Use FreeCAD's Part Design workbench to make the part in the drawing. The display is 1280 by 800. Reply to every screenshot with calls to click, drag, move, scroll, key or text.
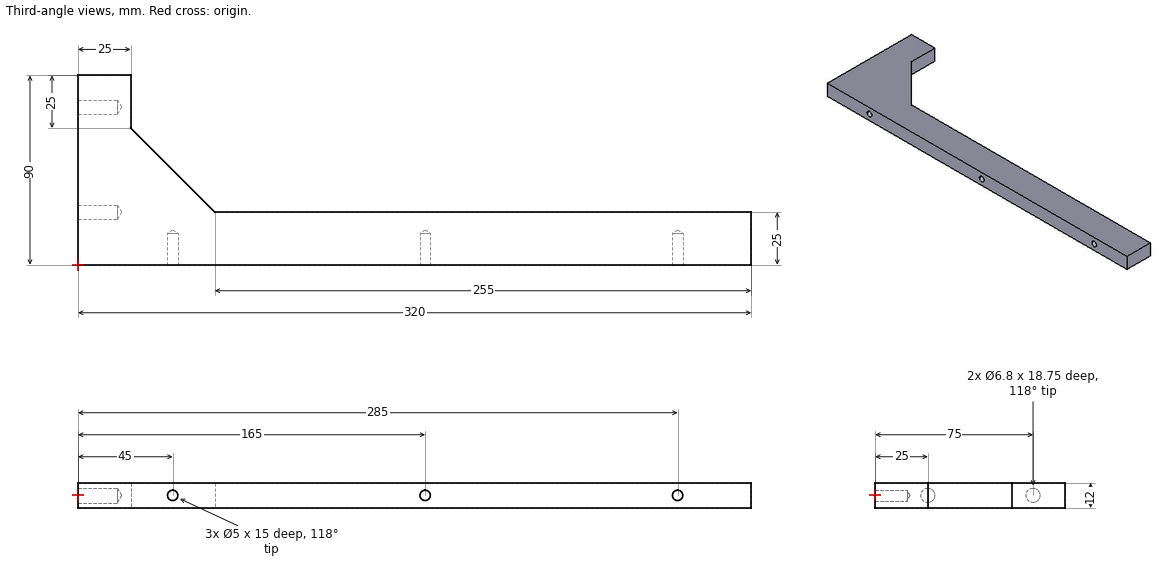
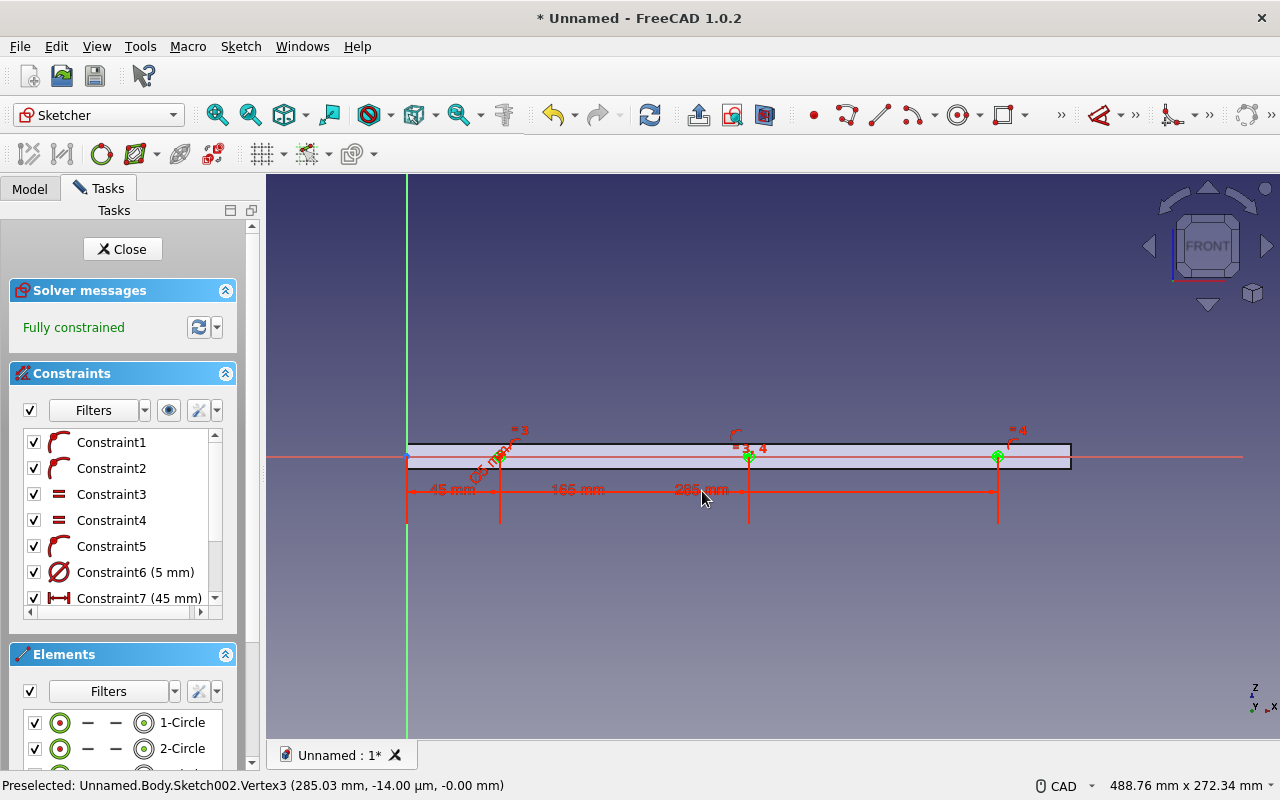
click(123, 249)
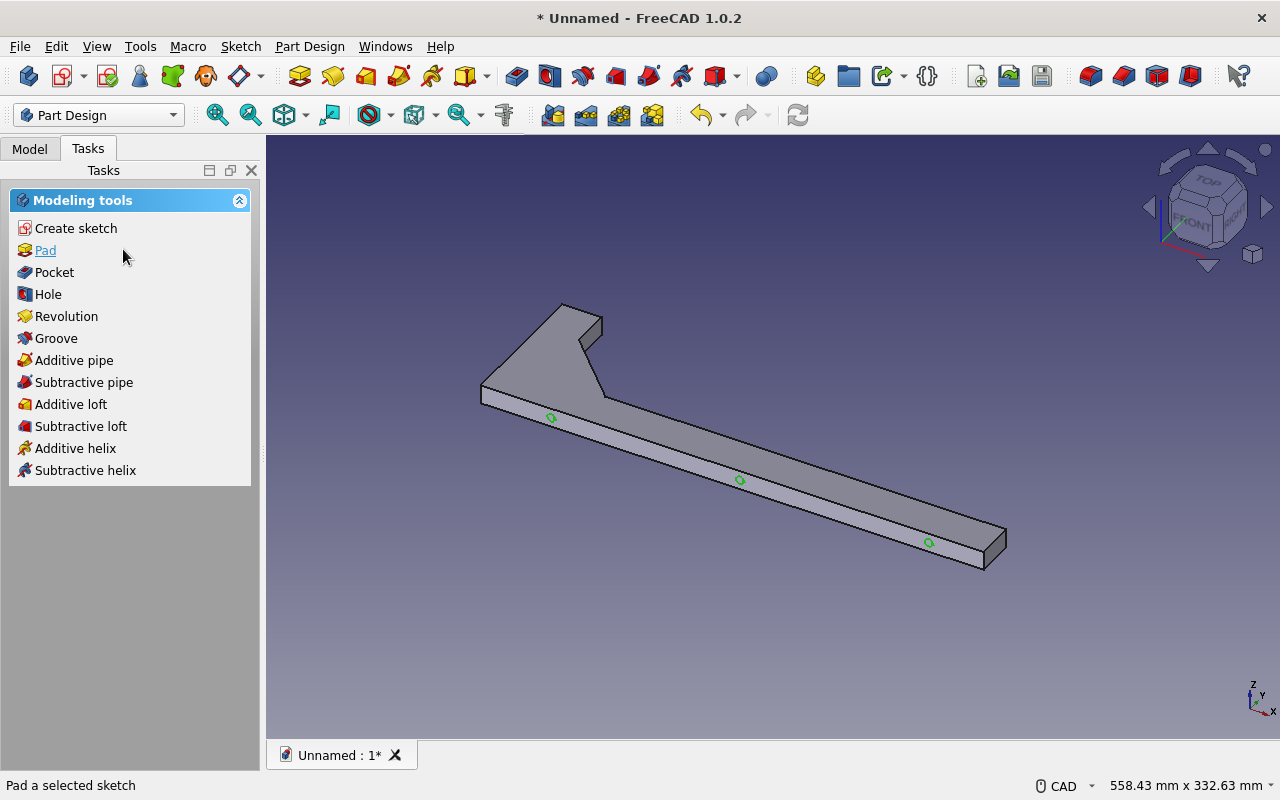
click(550, 76)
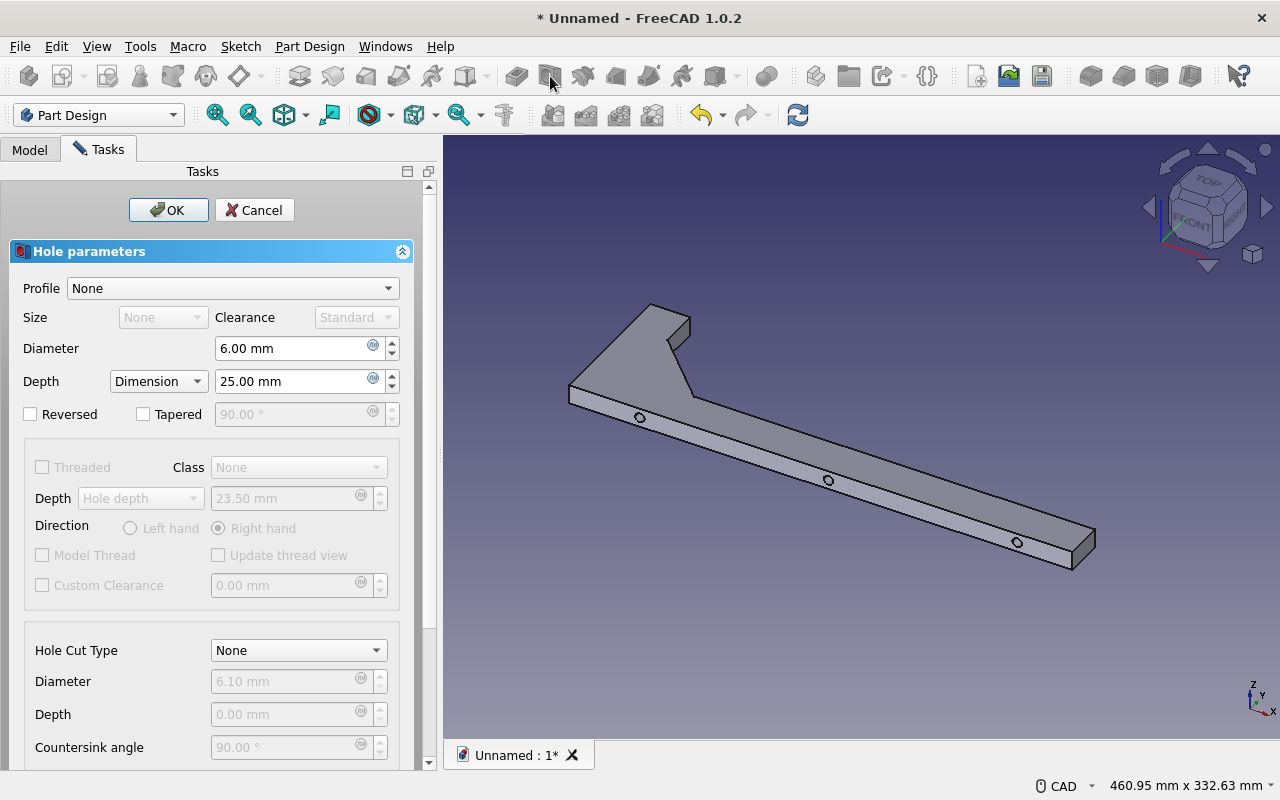
triple_click(300, 348)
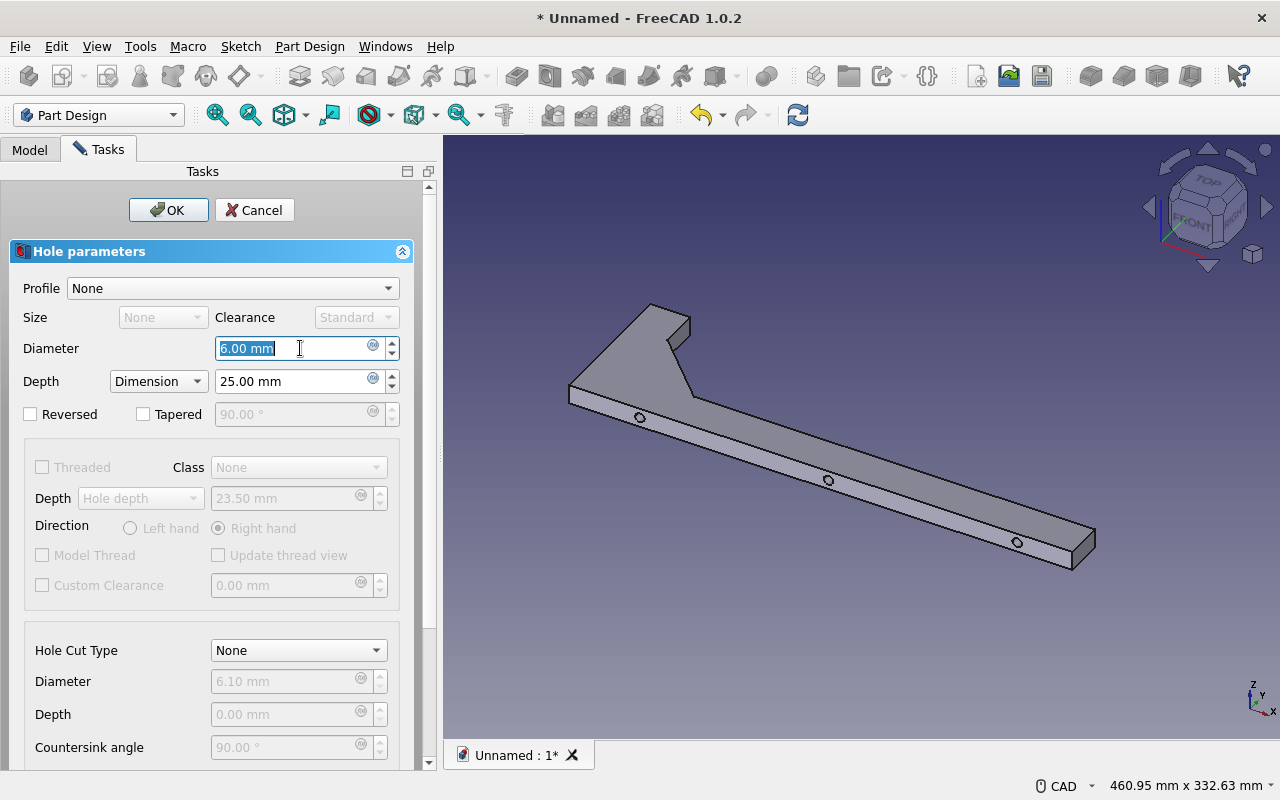
text(5)
key(Tab)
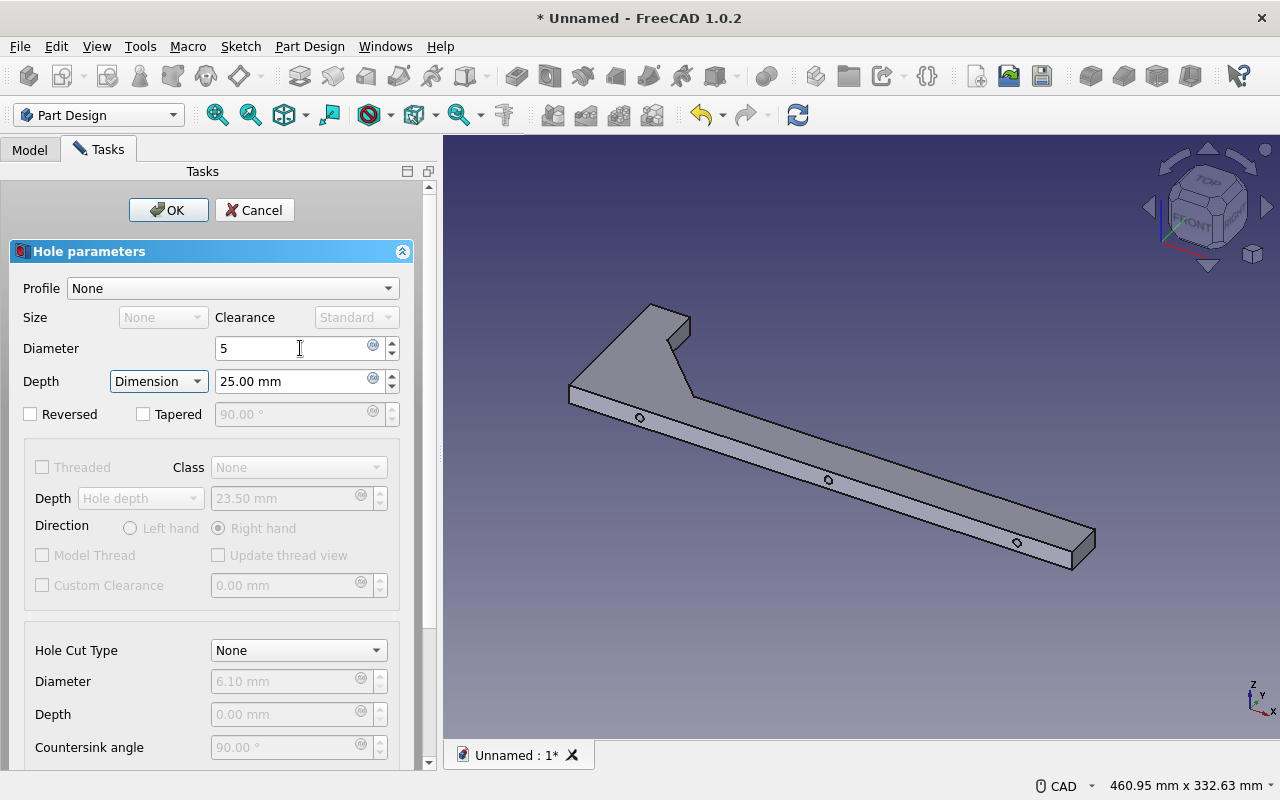
triple_click(300, 382)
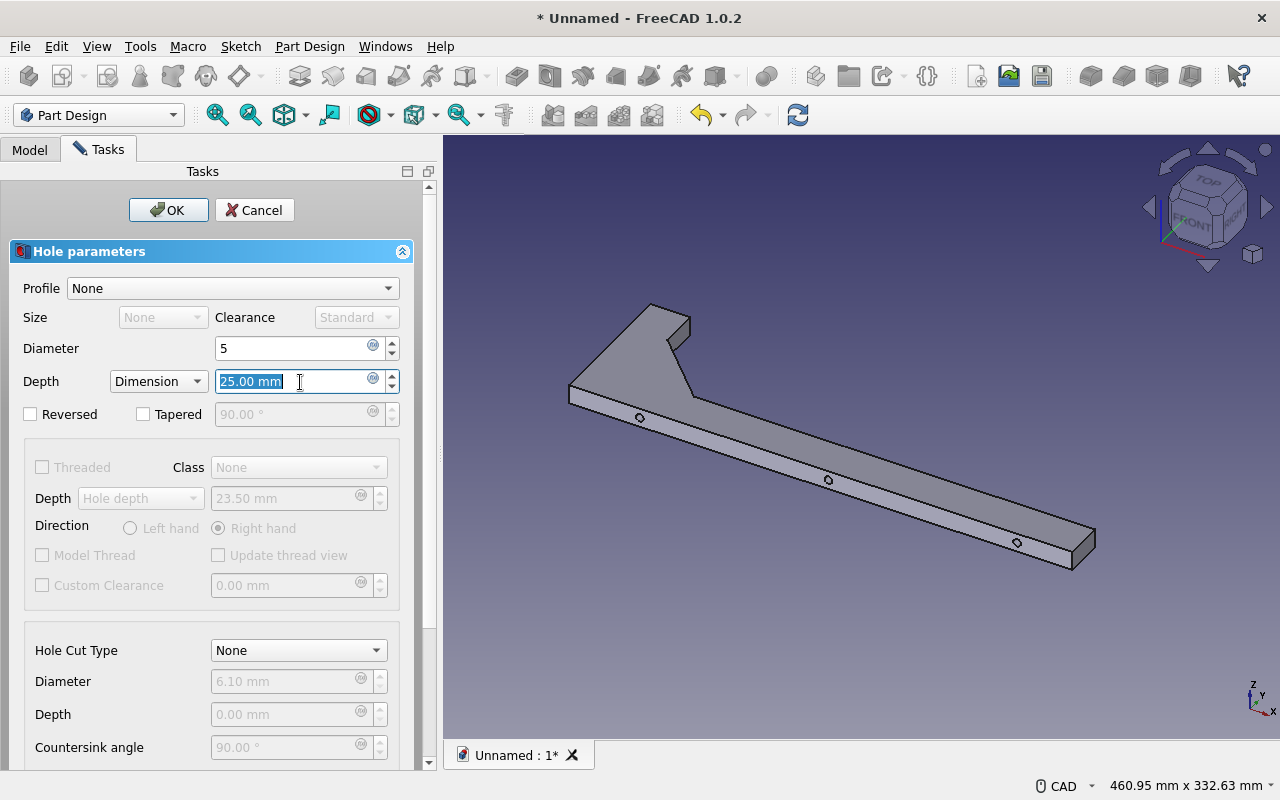
text(15)
key(Tab)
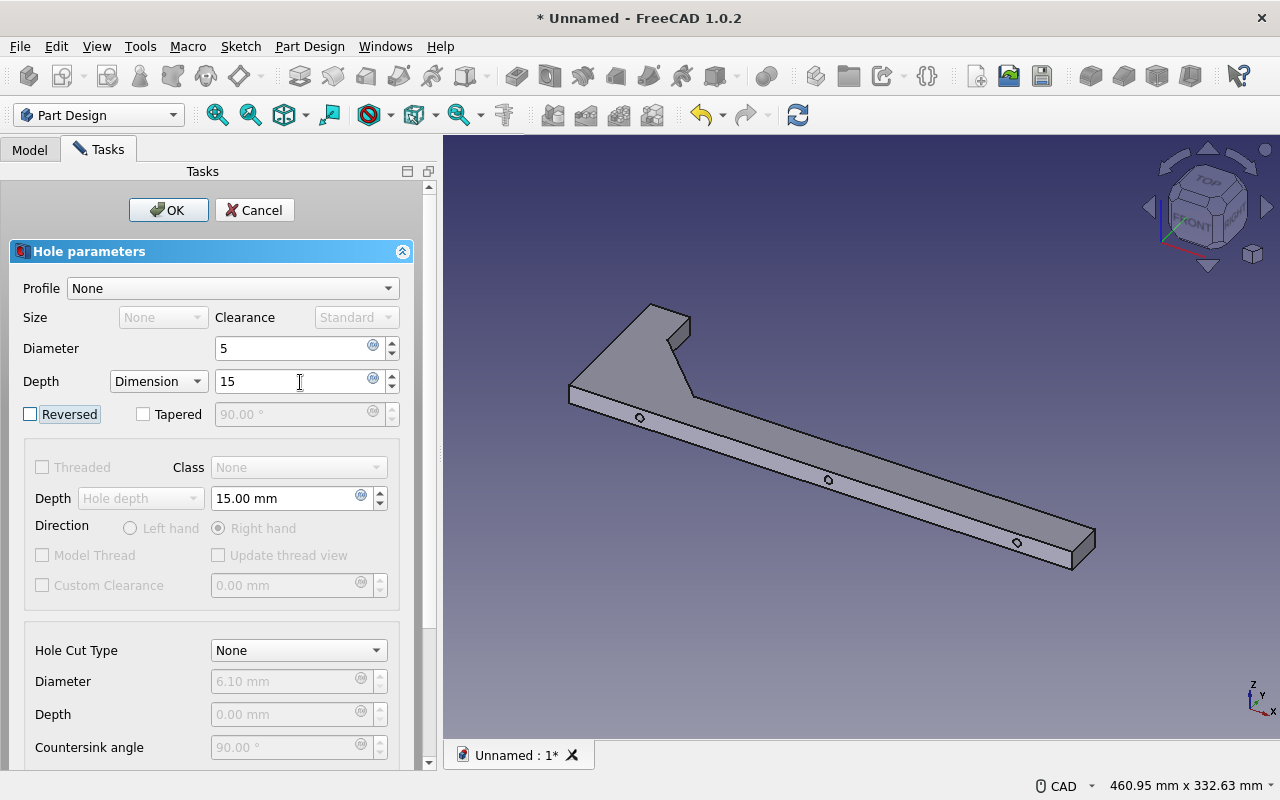
click(169, 210)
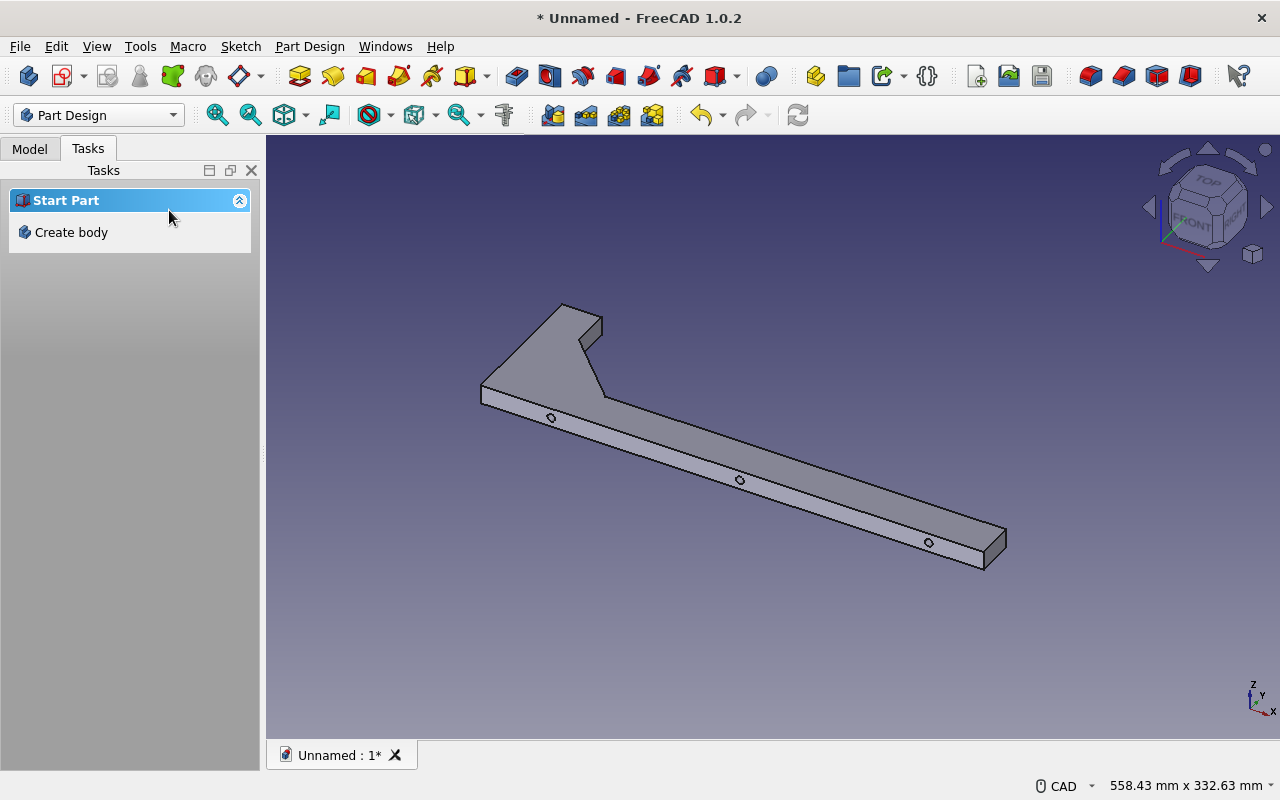
key(0)